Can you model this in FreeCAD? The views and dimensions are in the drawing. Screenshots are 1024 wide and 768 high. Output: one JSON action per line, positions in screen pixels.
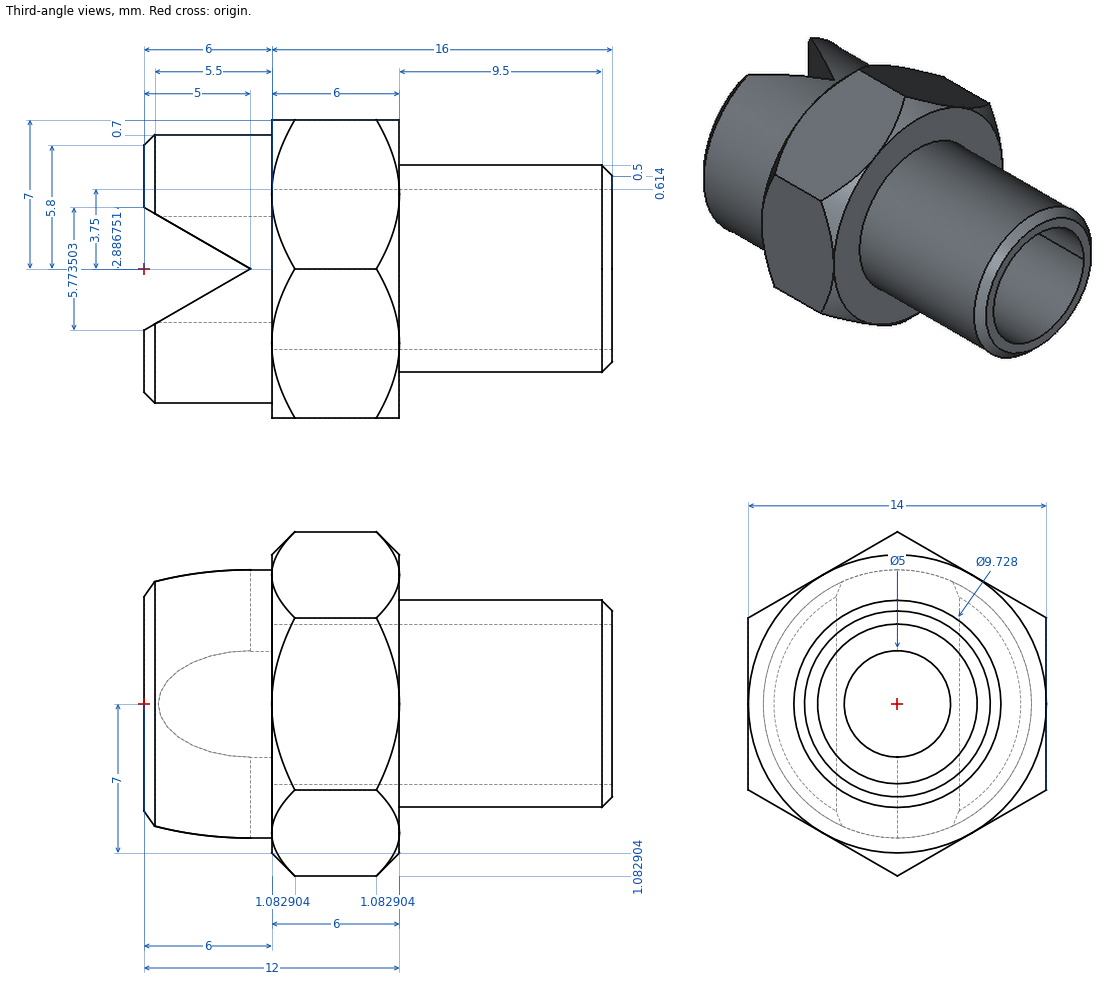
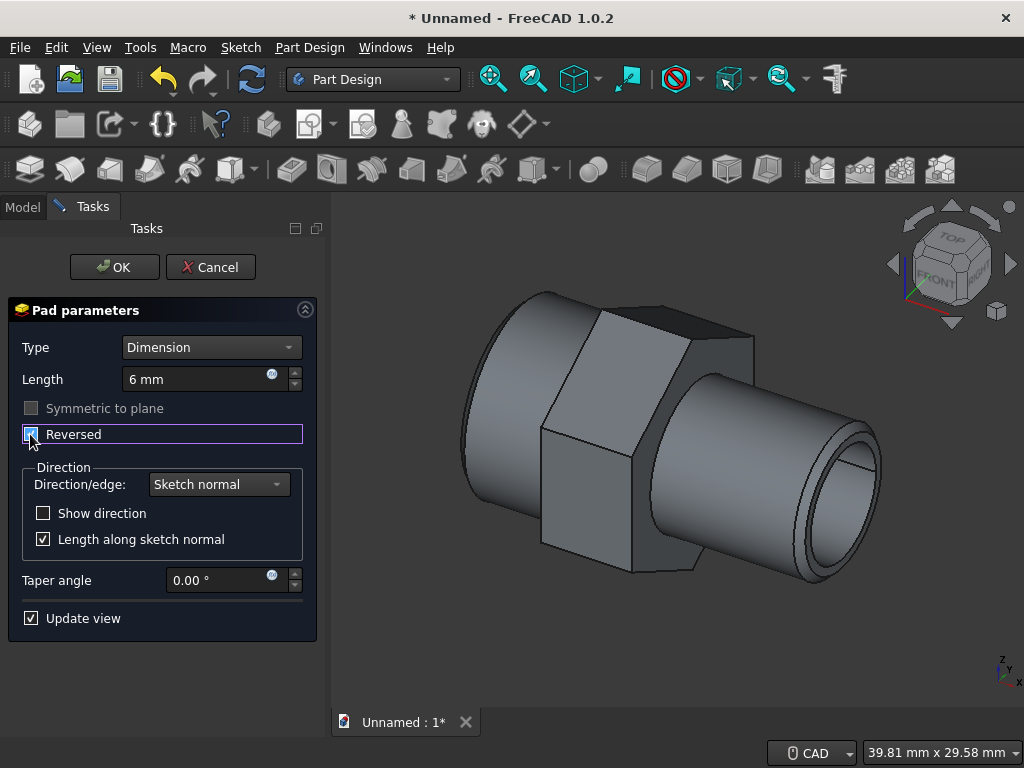
{"action": "left_click", "coordinate": [115, 267]}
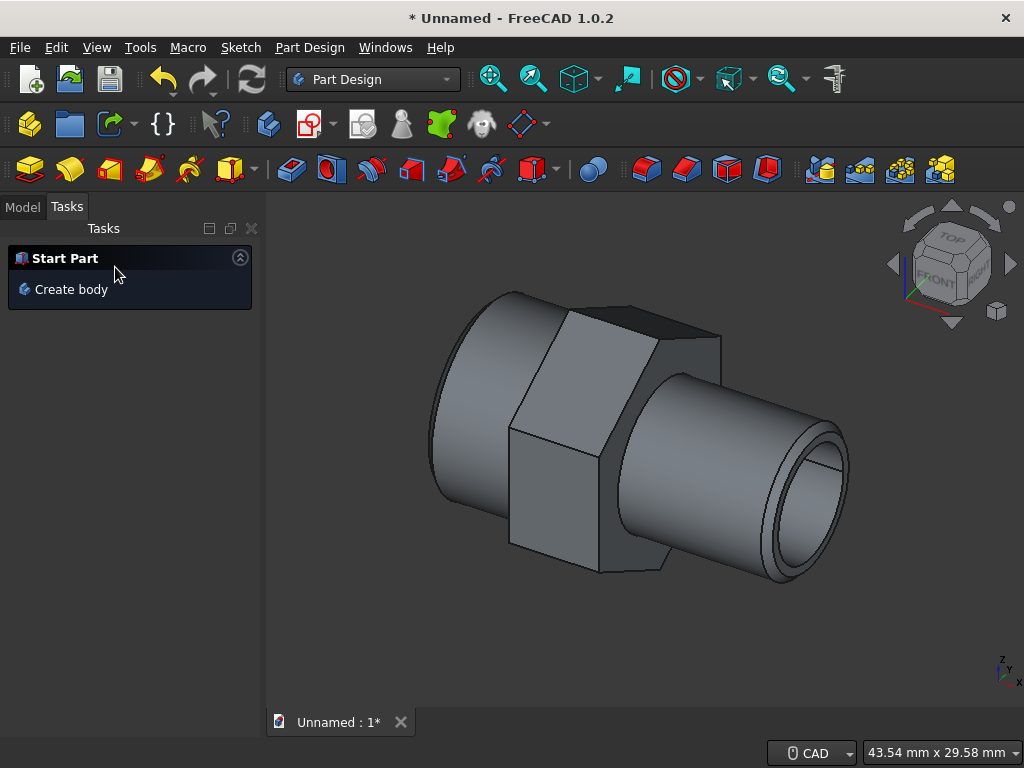
{"action": "left_click", "coordinate": [310, 124]}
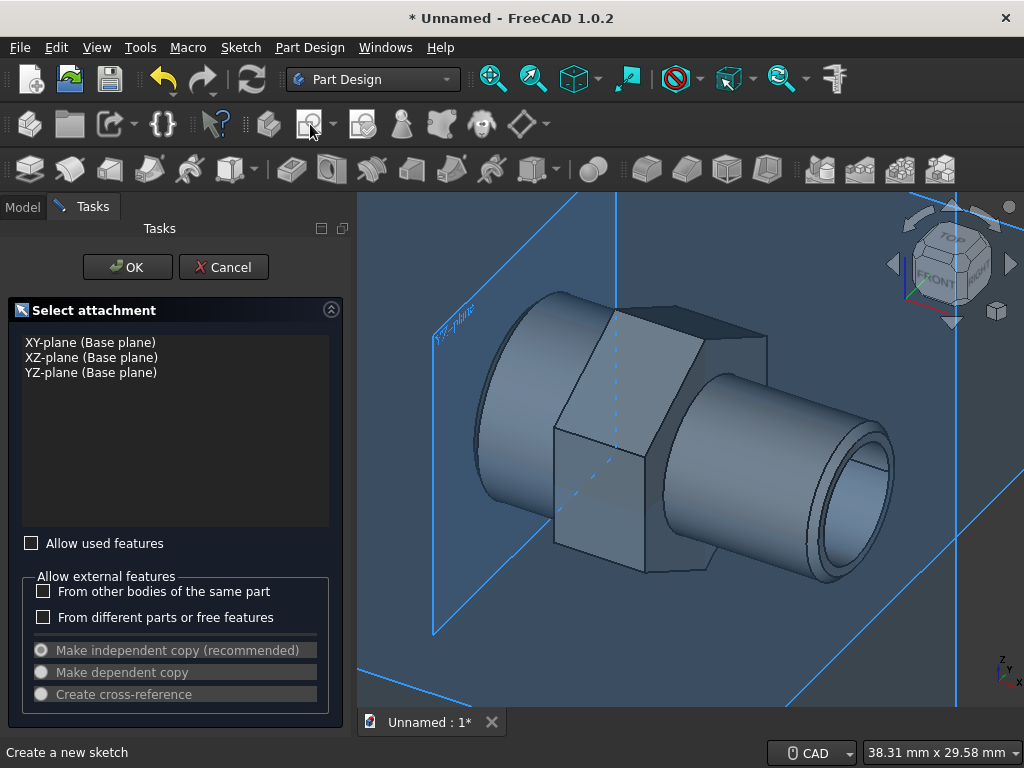
{"action": "left_click", "coordinate": [82, 358]}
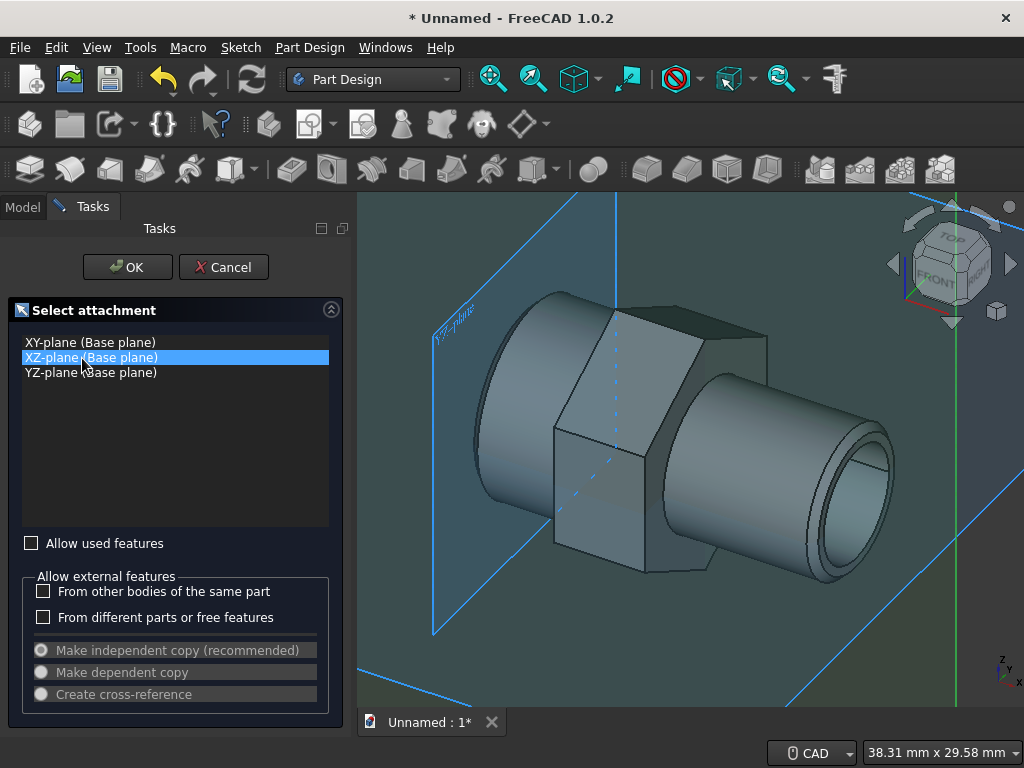
{"action": "left_click", "coordinate": [128, 267]}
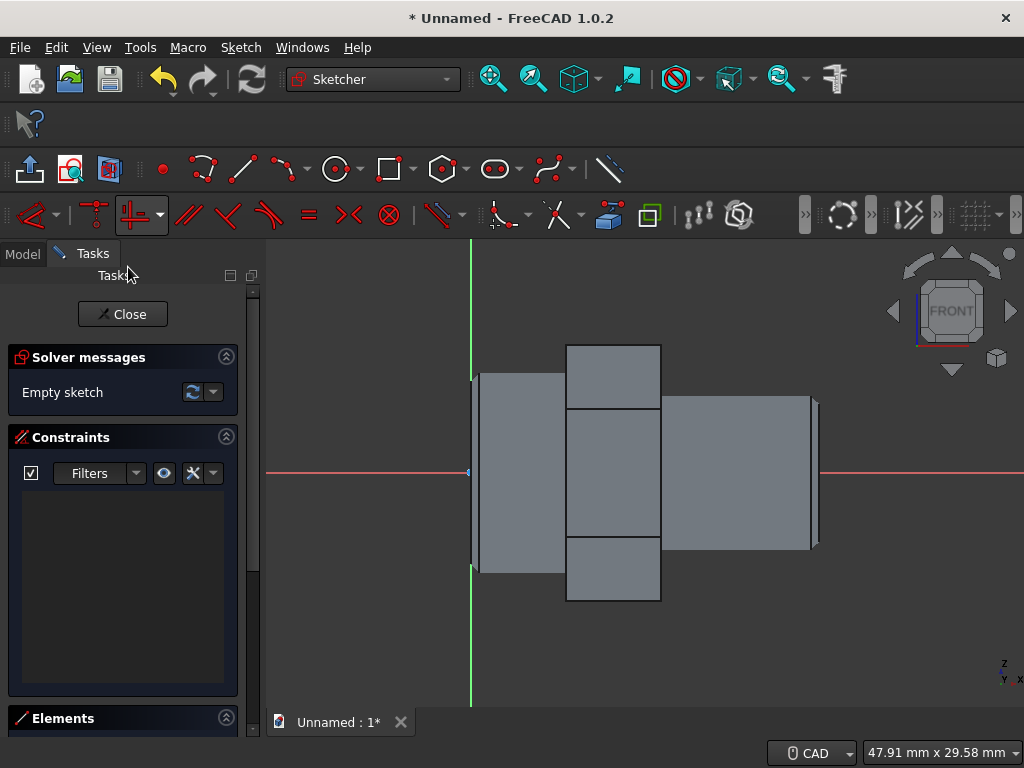
{"action": "left_click", "coordinate": [110, 170]}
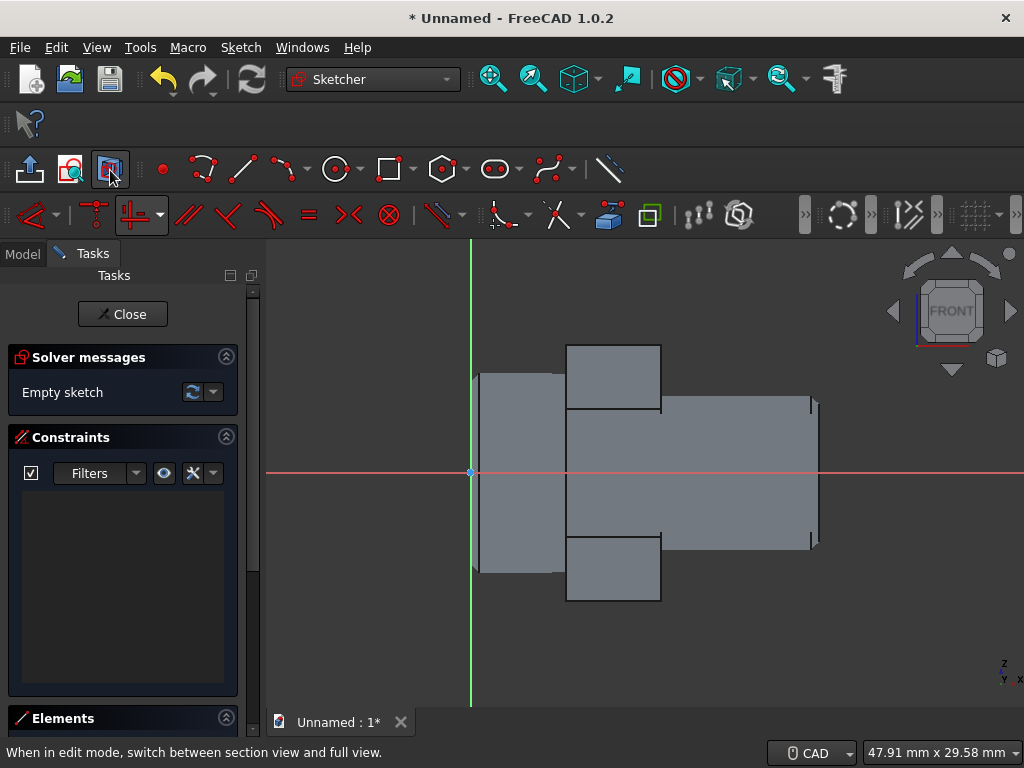
{"action": "scroll", "coordinate": [557, 589], "scroll_direction": "up", "scroll_amount": 4}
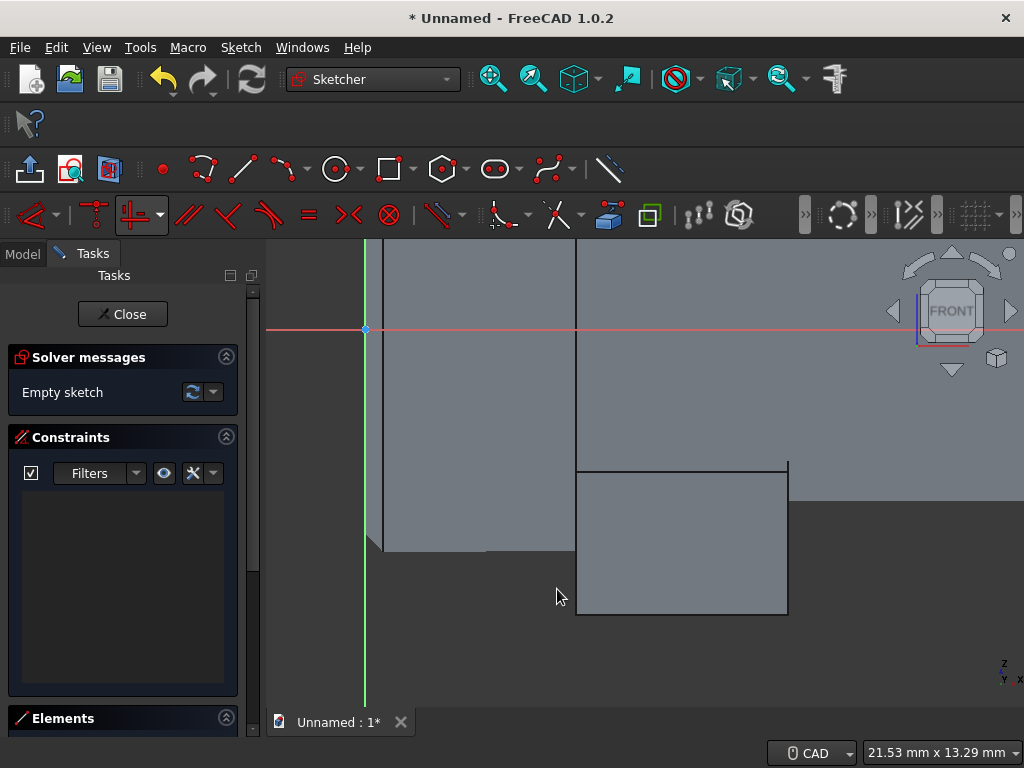
{"action": "left_click", "coordinate": [204, 170]}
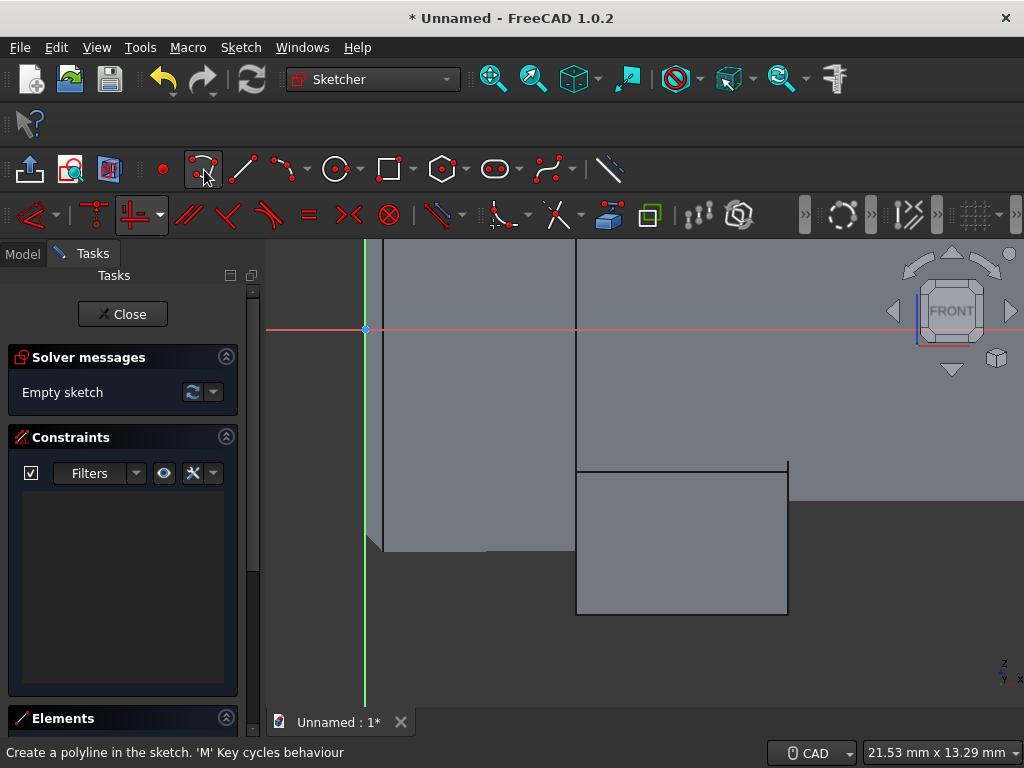
{"action": "left_click", "coordinate": [749, 615]}
{"action": "left_click", "coordinate": [788, 576]}
{"action": "left_click", "coordinate": [788, 615]}
{"action": "left_click", "coordinate": [749, 616]}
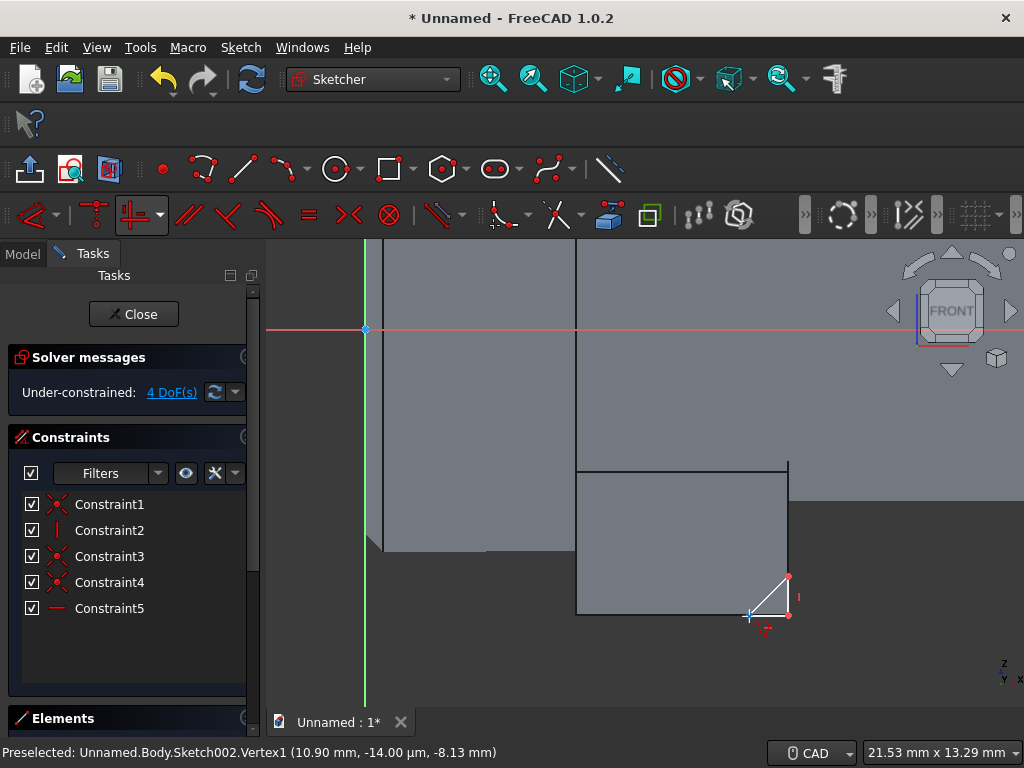
{"action": "left_click", "coordinate": [576, 576]}
{"action": "left_click", "coordinate": [614, 615]}
{"action": "left_click", "coordinate": [576, 615]}
{"action": "left_click", "coordinate": [576, 577]}
{"action": "key", "text": "Escape"}
{"action": "key", "text": "Escape"}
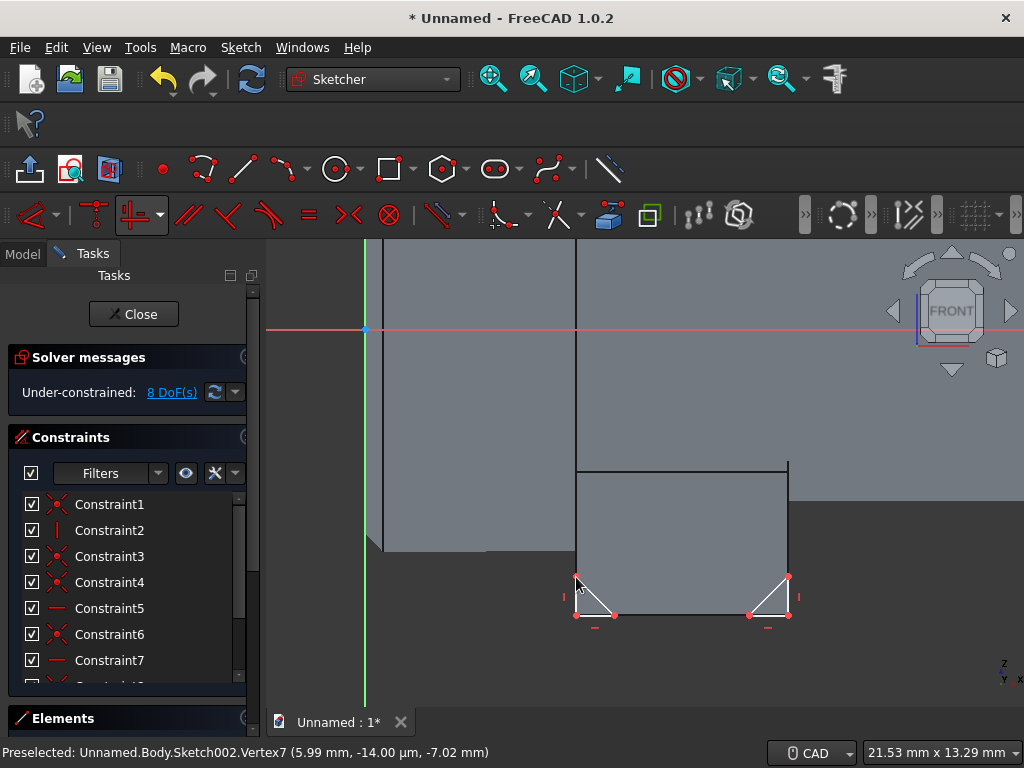
{"action": "left_click", "coordinate": [32, 216]}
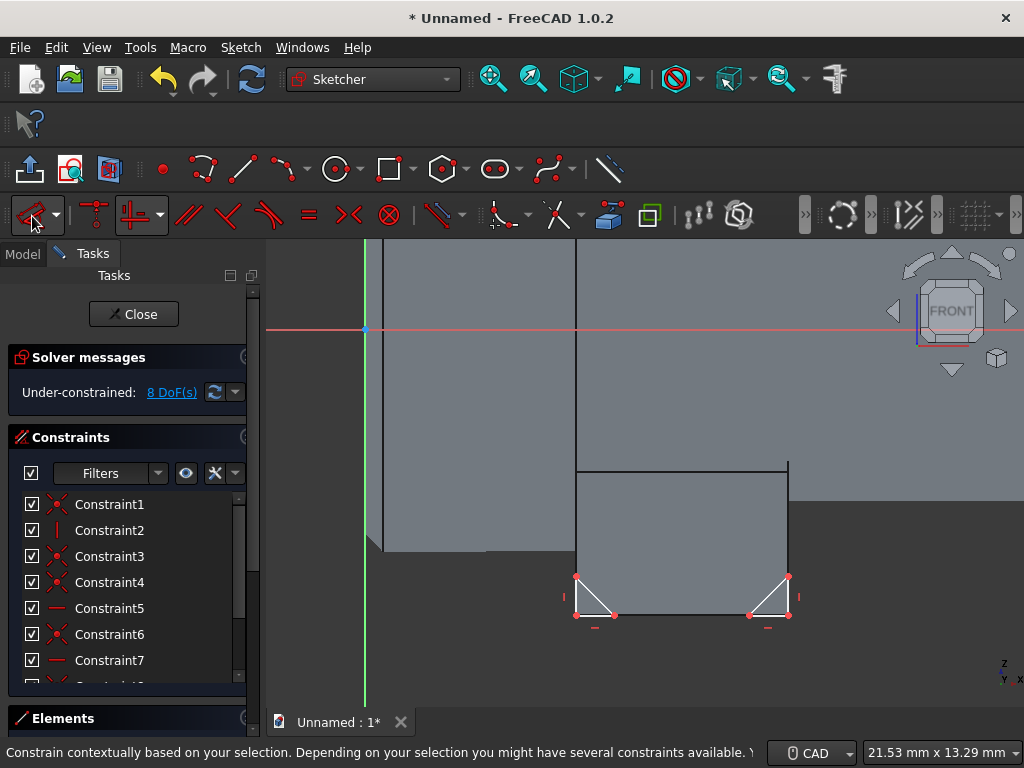
{"action": "left_click", "coordinate": [788, 577]}
{"action": "left_click", "coordinate": [822, 453]}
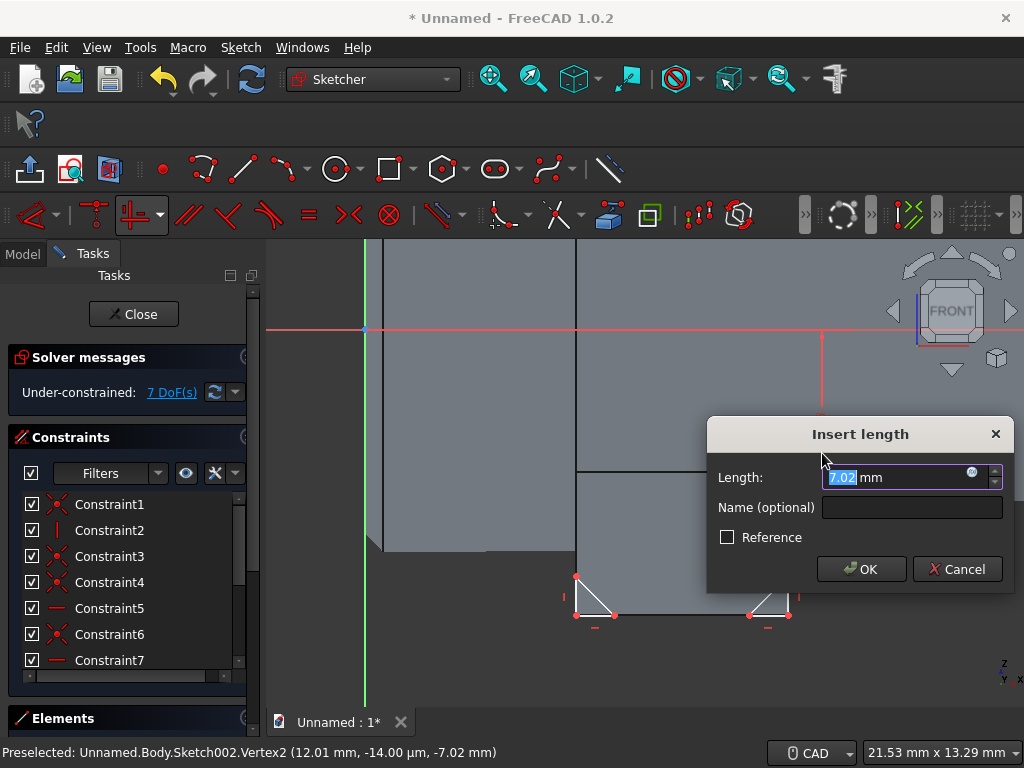
{"action": "type", "text": "7"}
{"action": "key", "text": "Return"}